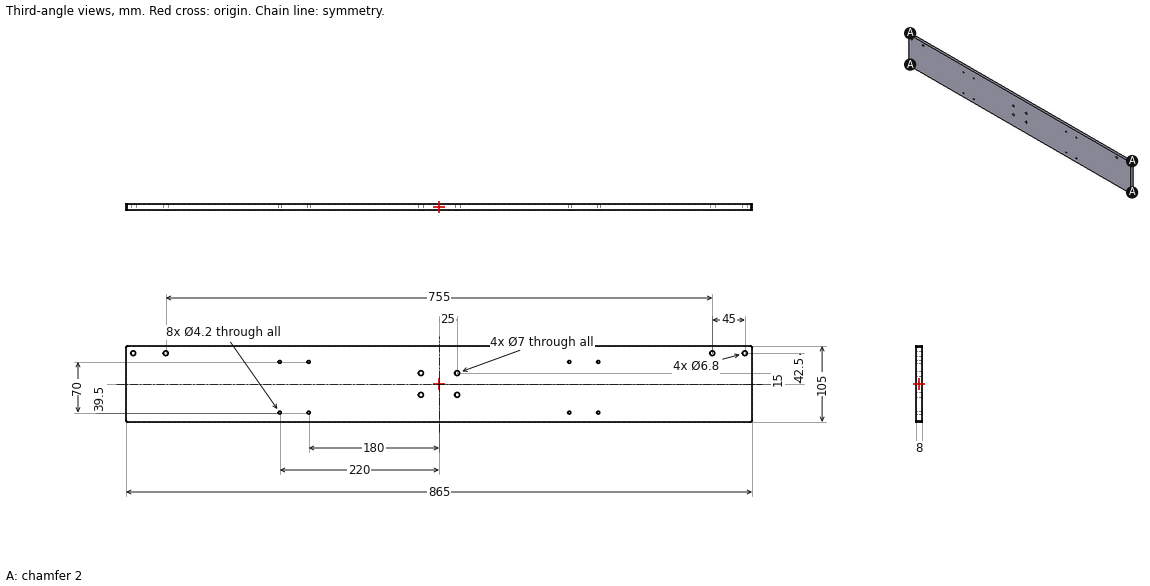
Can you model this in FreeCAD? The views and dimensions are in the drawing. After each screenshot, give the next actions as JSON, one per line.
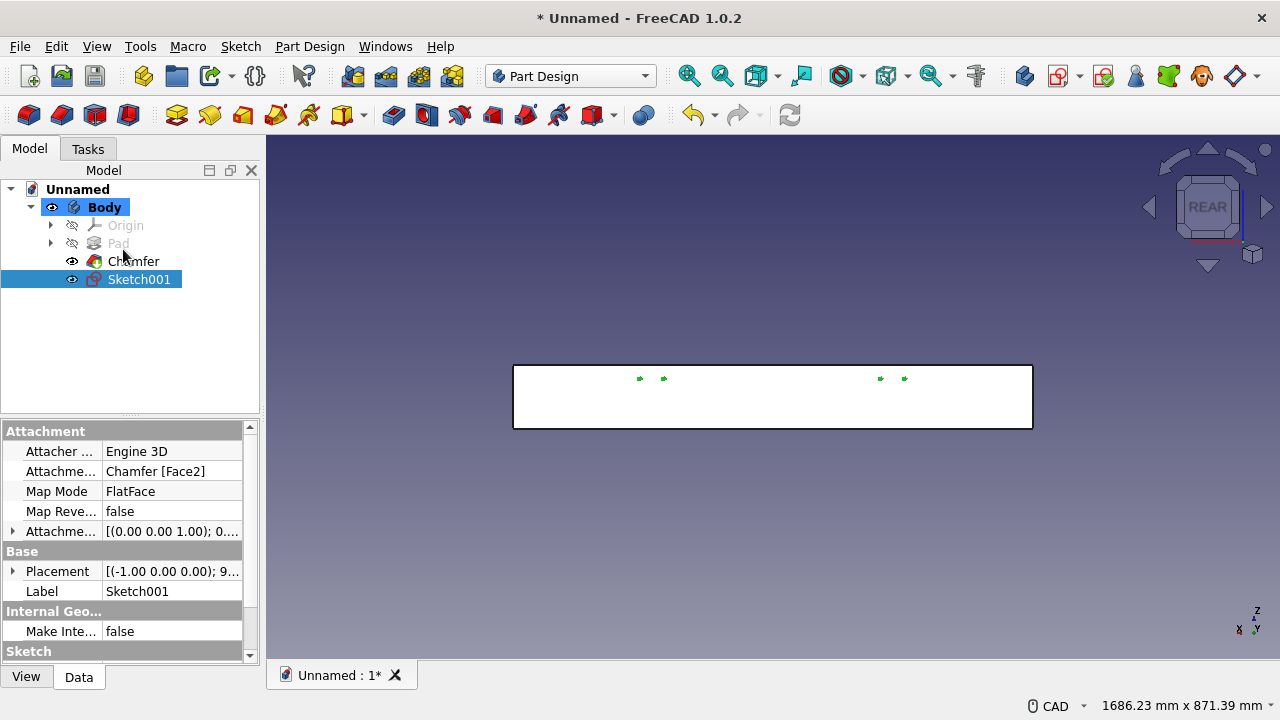
{"action": "left_click", "coordinate": [427, 116]}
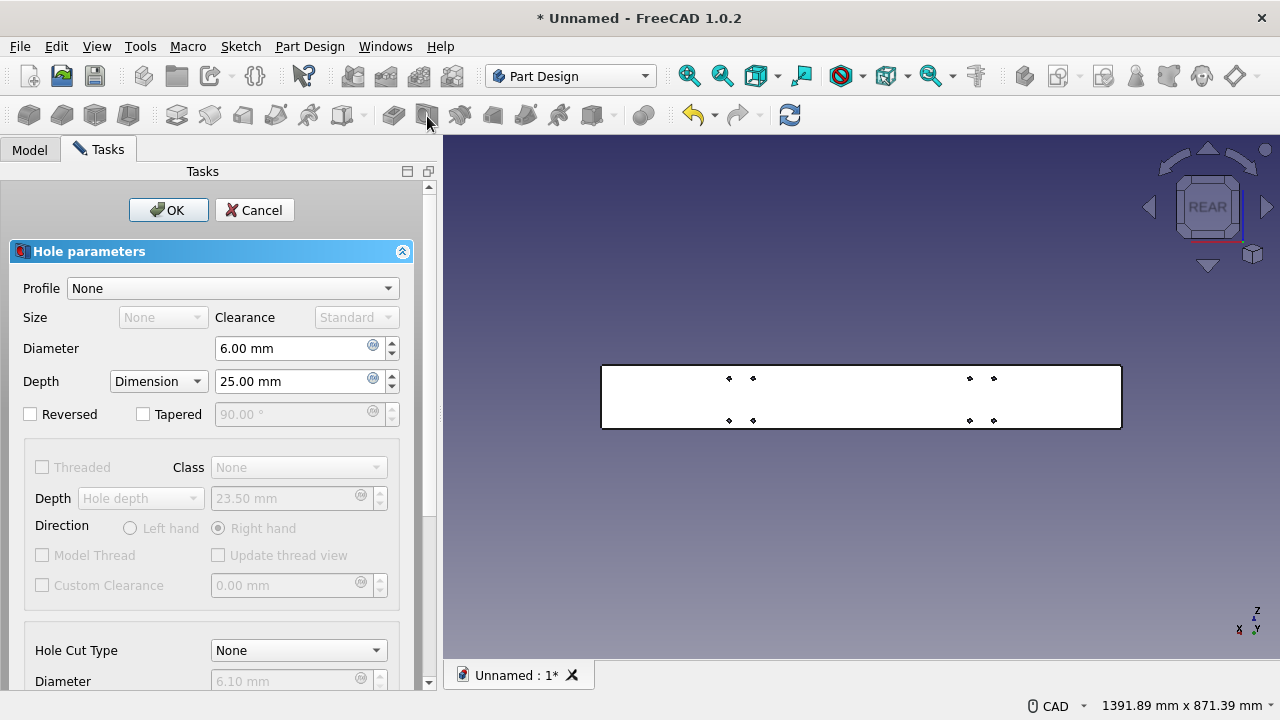
{"action": "triple_click", "coordinate": [300, 348]}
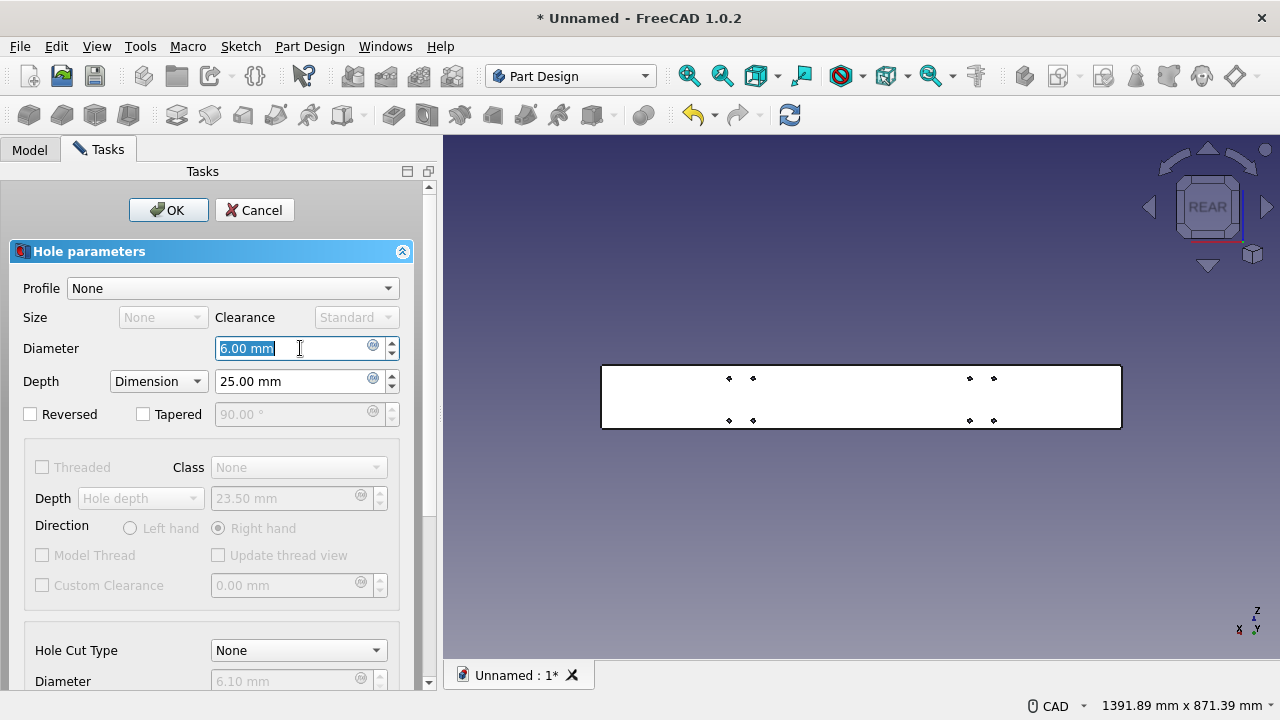
{"action": "type", "text": "4.2"}
{"action": "key", "text": "Tab"}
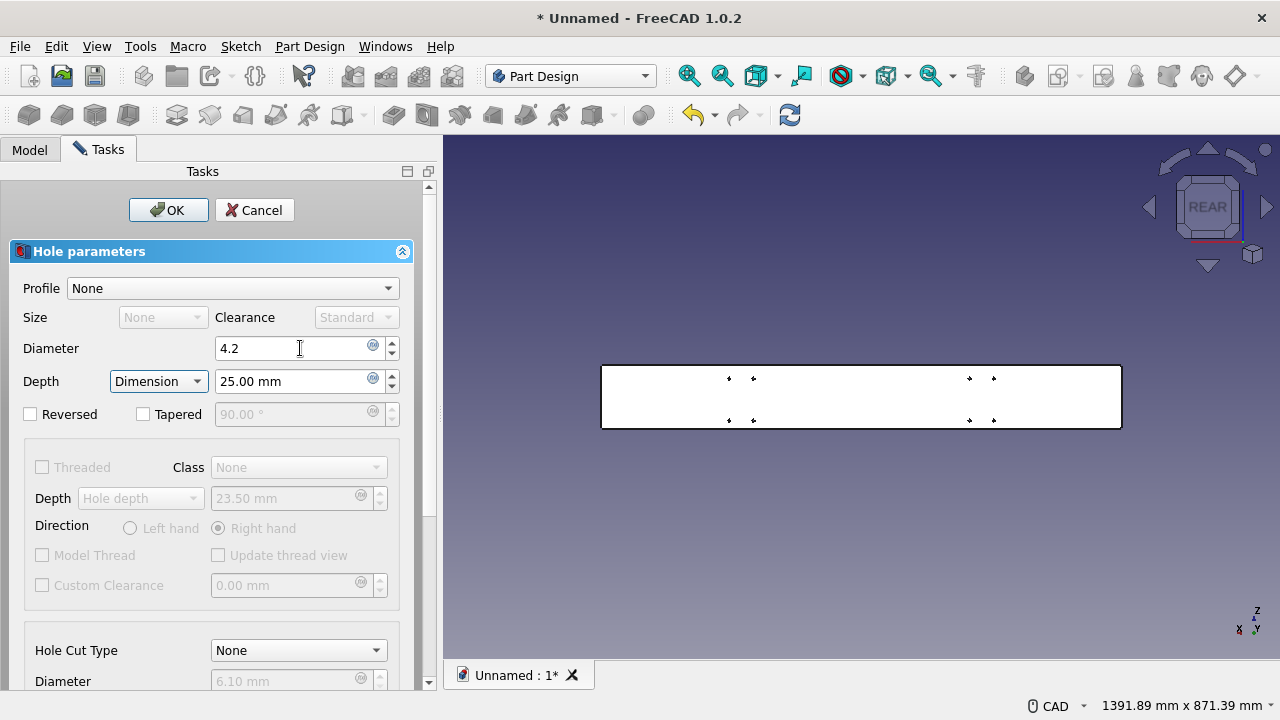
{"action": "left_click", "coordinate": [160, 382]}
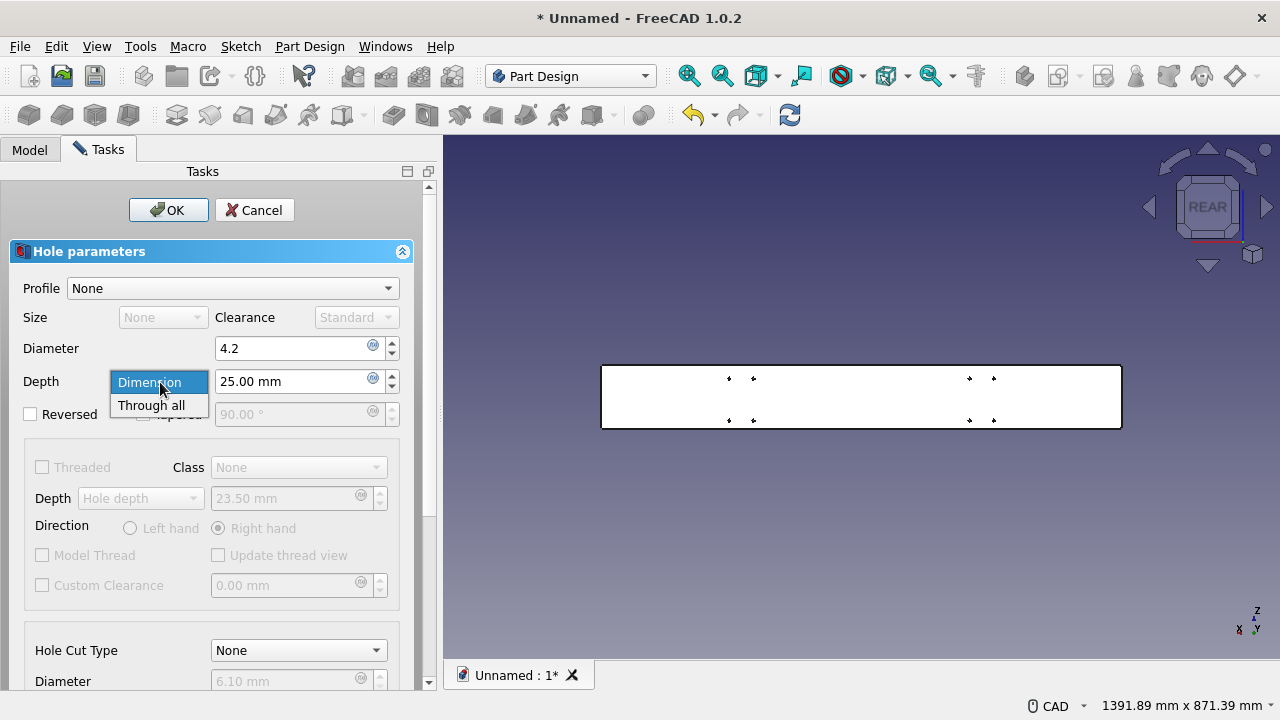
{"action": "left_click", "coordinate": [158, 406]}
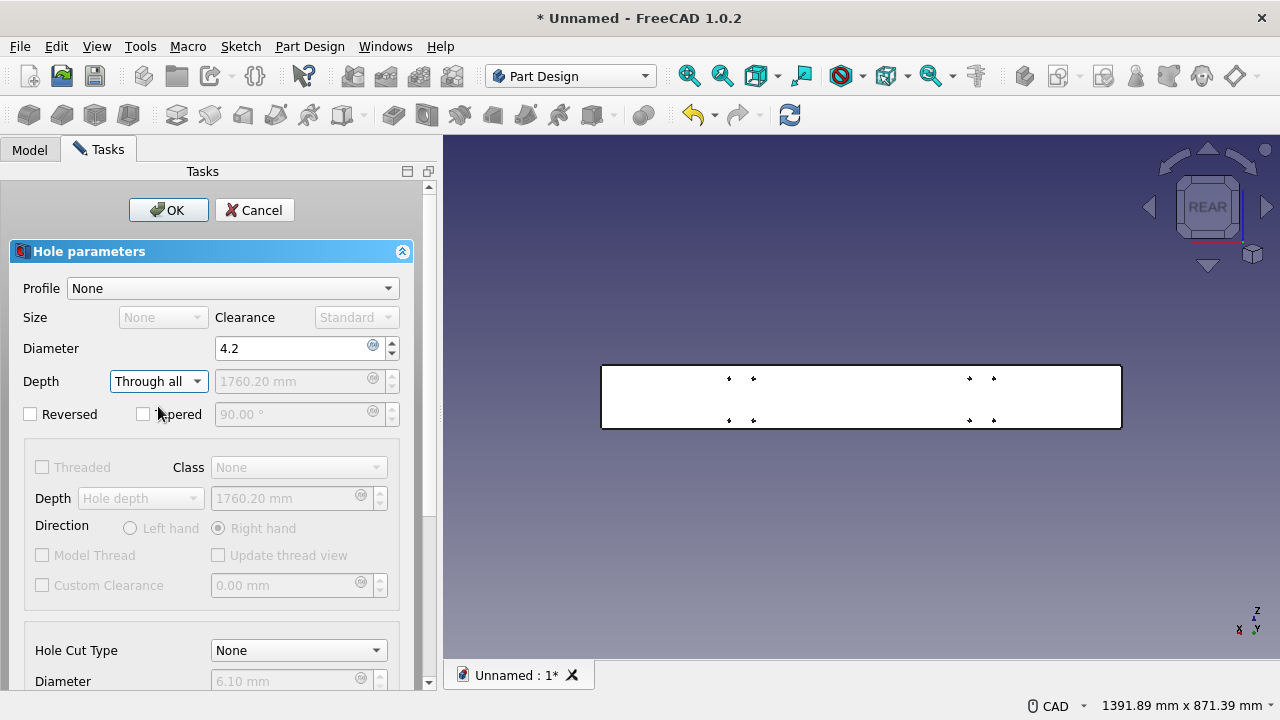
{"action": "left_click", "coordinate": [169, 210]}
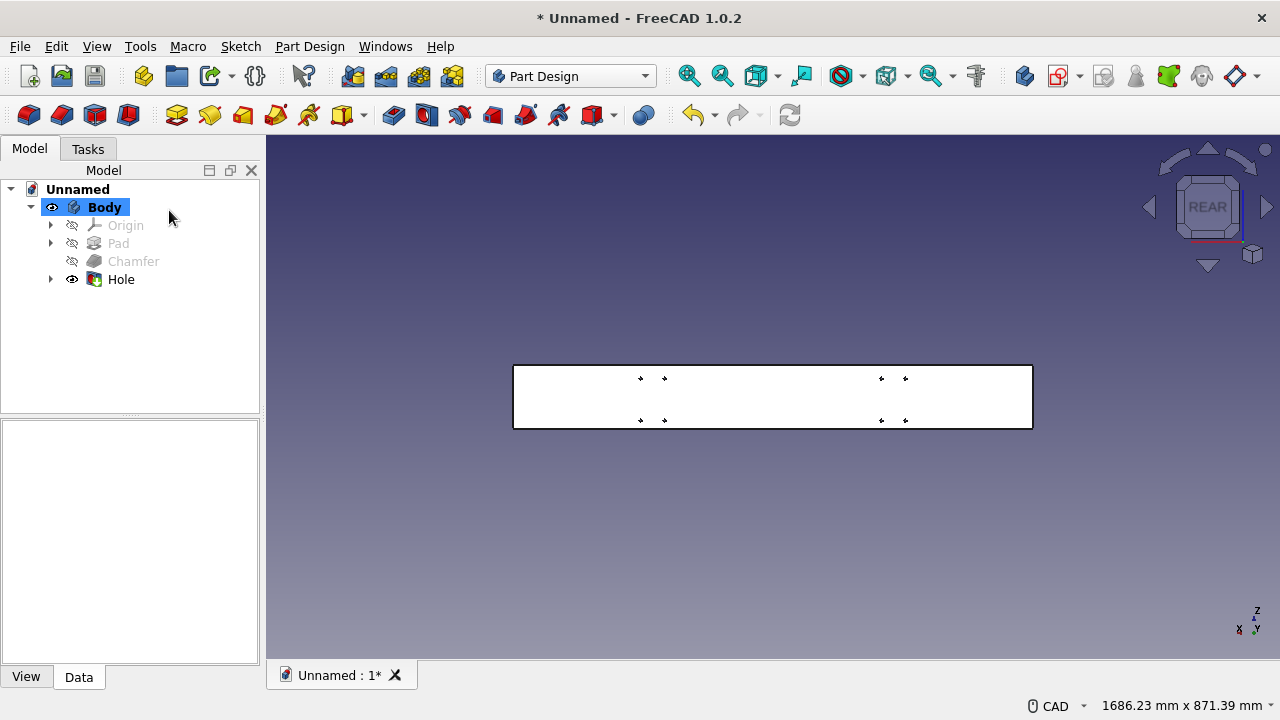
{"action": "left_click", "coordinate": [550, 396]}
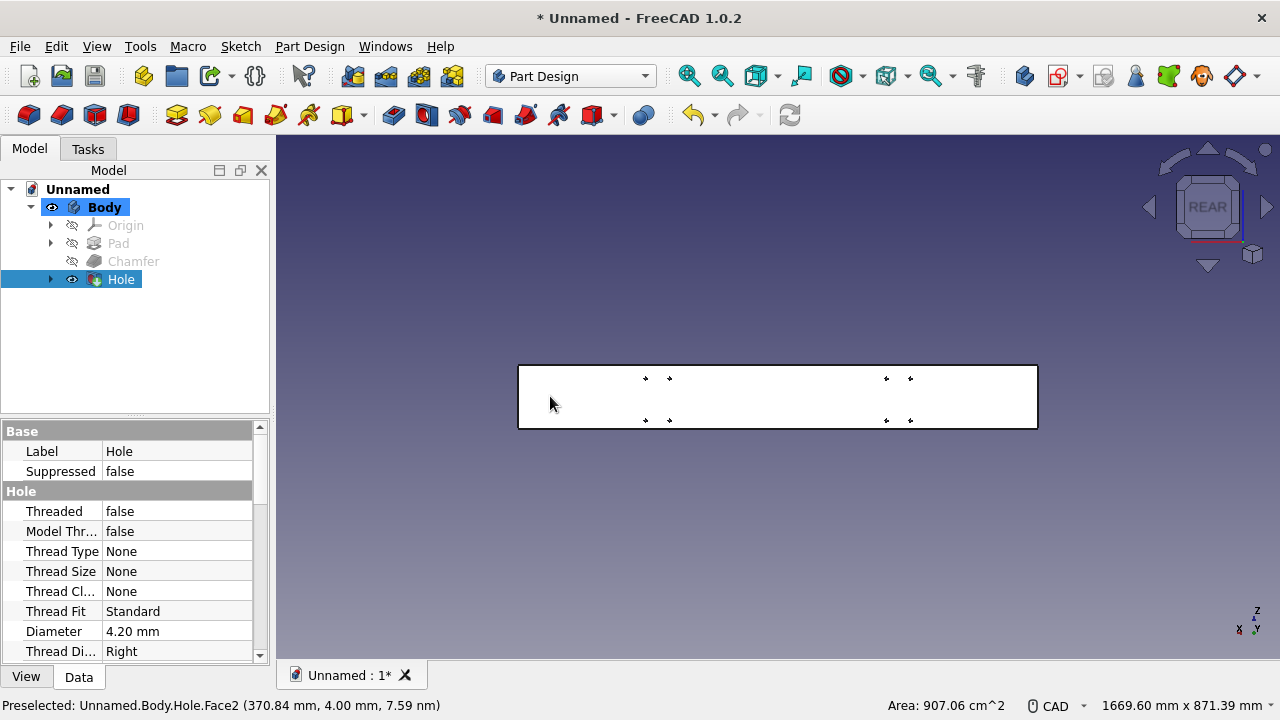
{"action": "left_click", "coordinate": [1058, 76]}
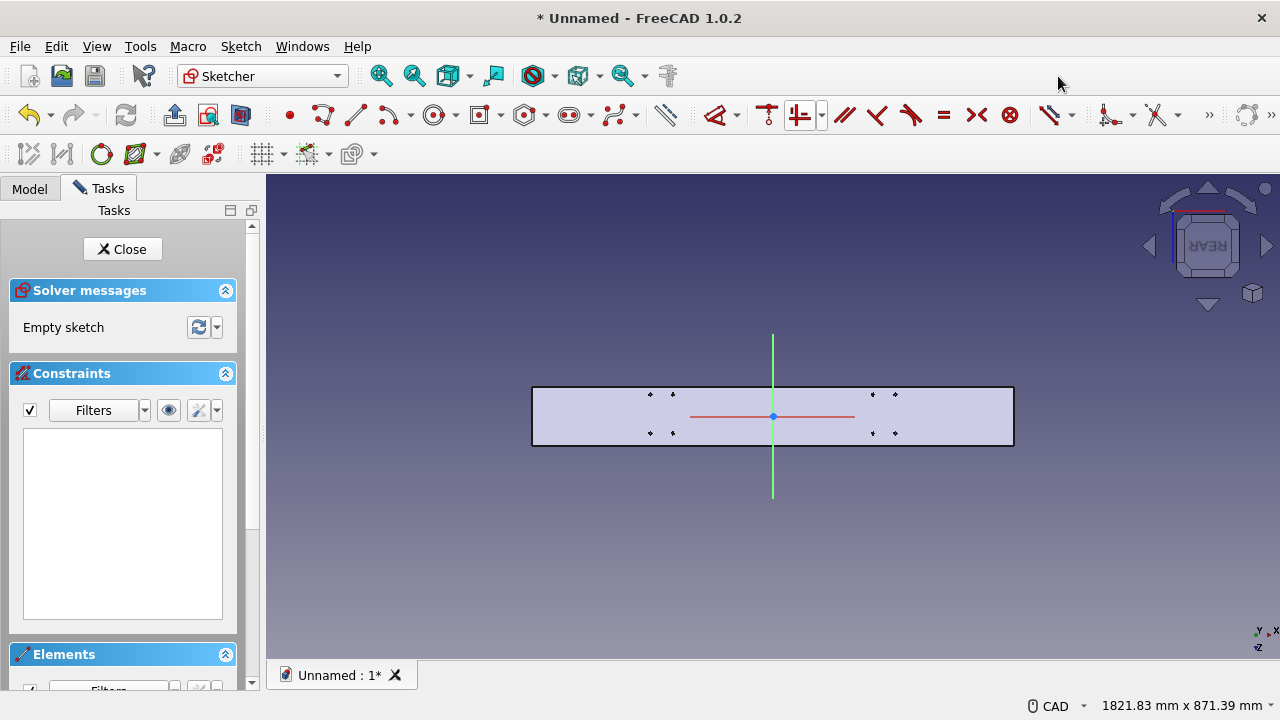
{"action": "scroll", "coordinate": [778, 416], "scroll_direction": "up", "scroll_amount": 13}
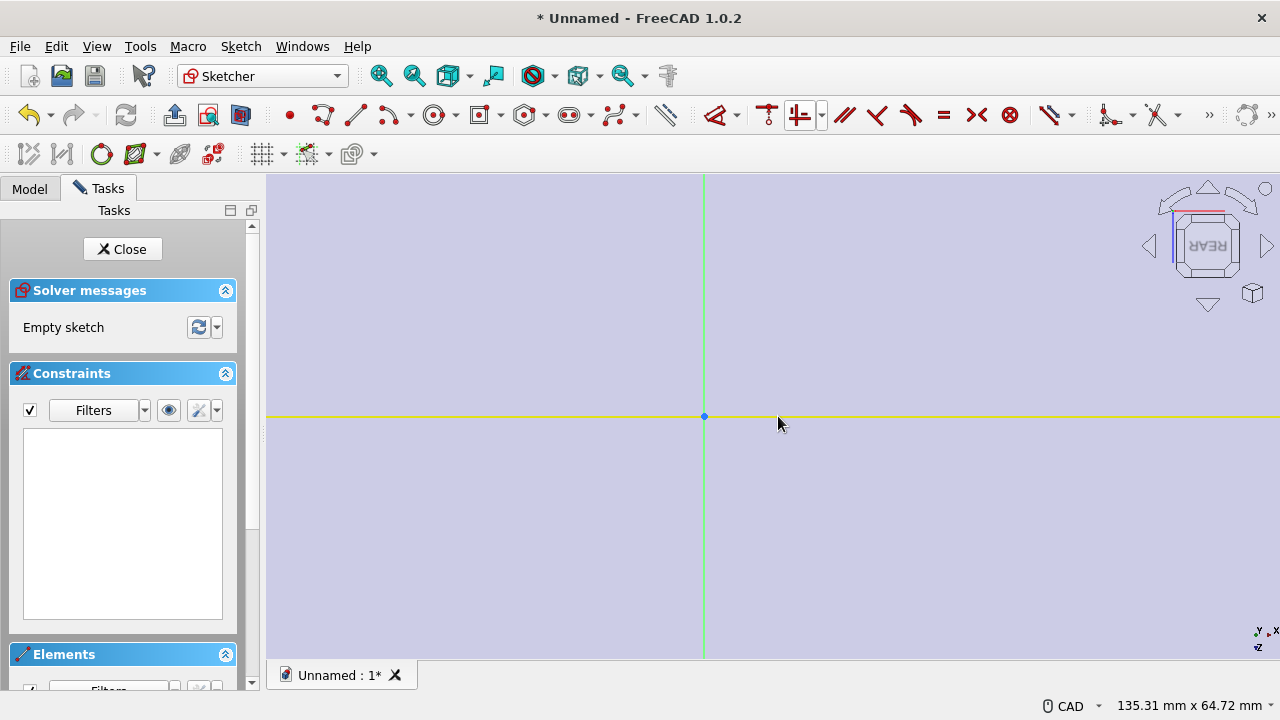
{"action": "left_click", "coordinate": [434, 116]}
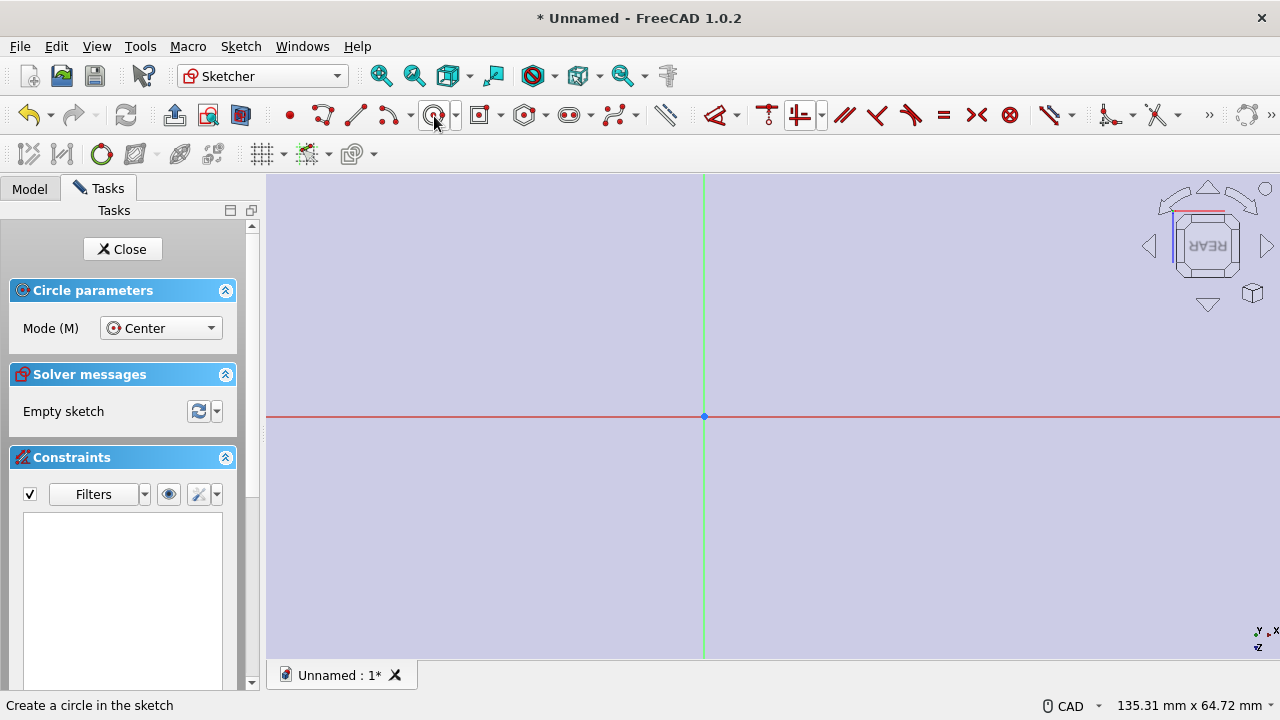
{"action": "left_click", "coordinate": [892, 529]}
{"action": "left_click", "coordinate": [910, 510]}